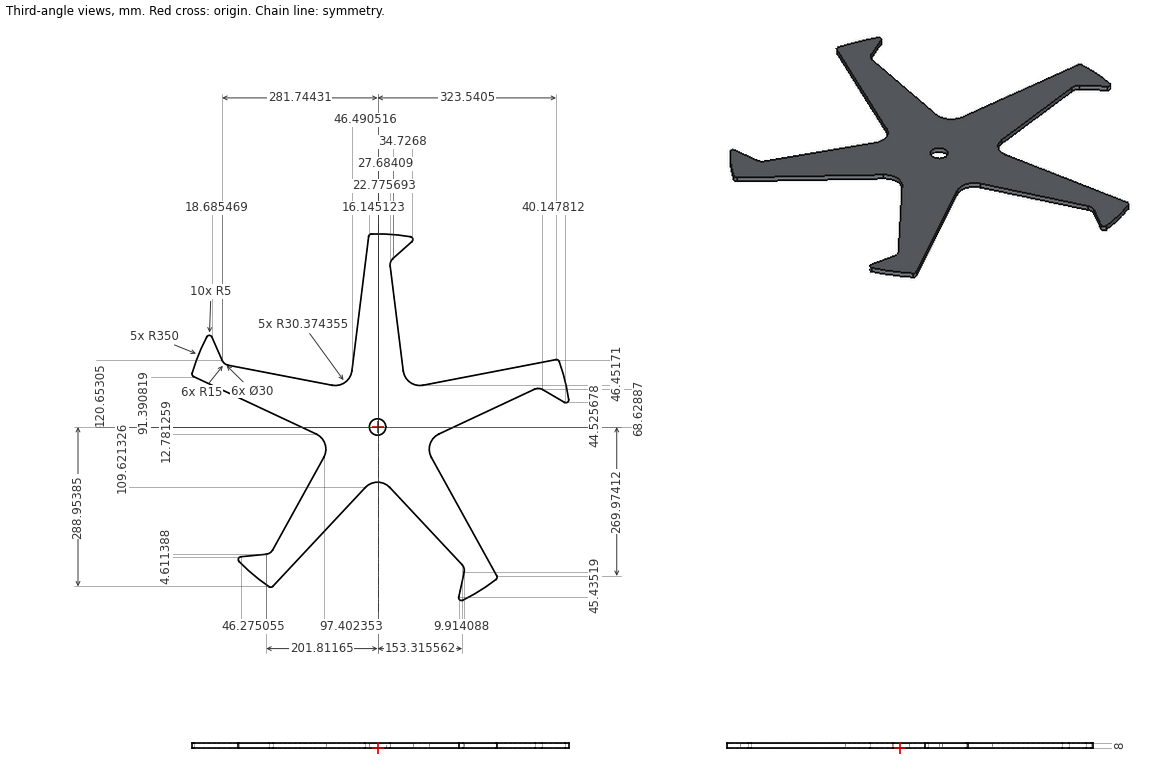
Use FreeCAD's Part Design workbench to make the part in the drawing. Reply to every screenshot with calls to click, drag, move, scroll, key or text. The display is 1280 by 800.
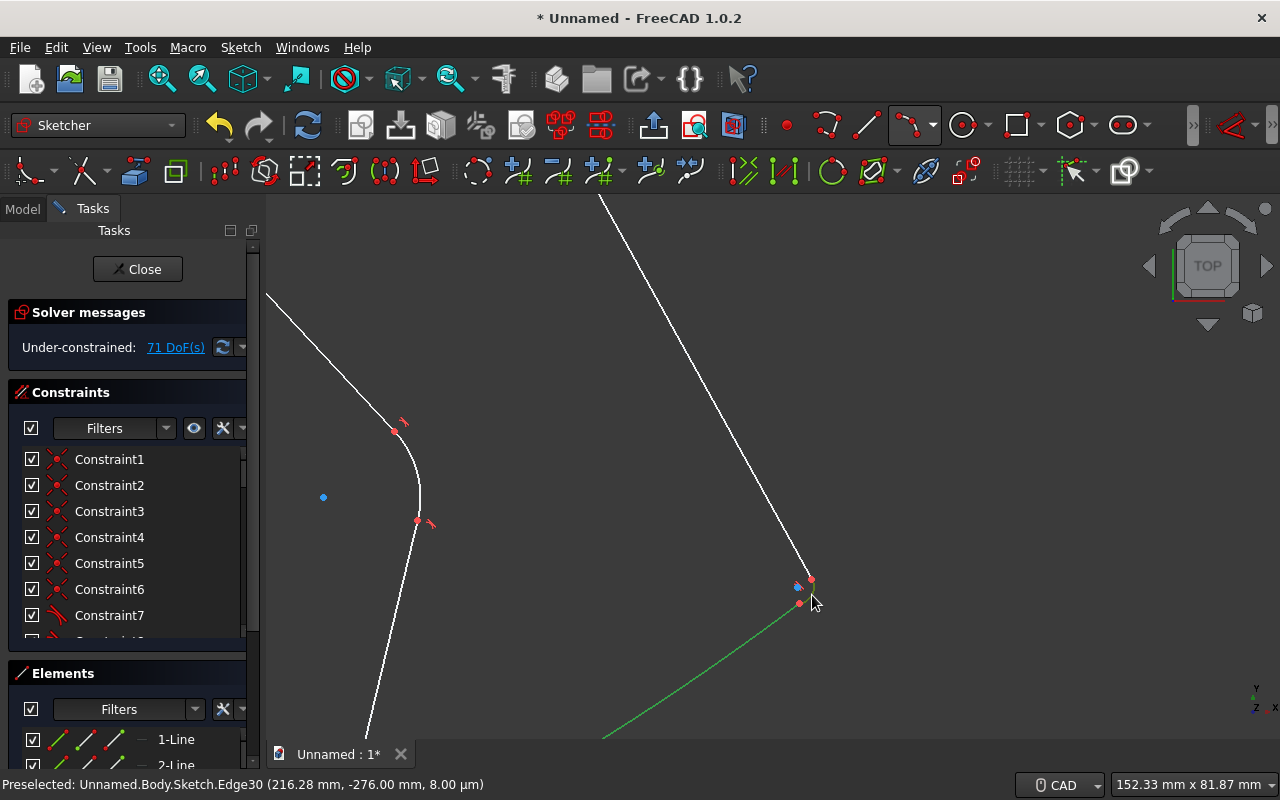
key(t)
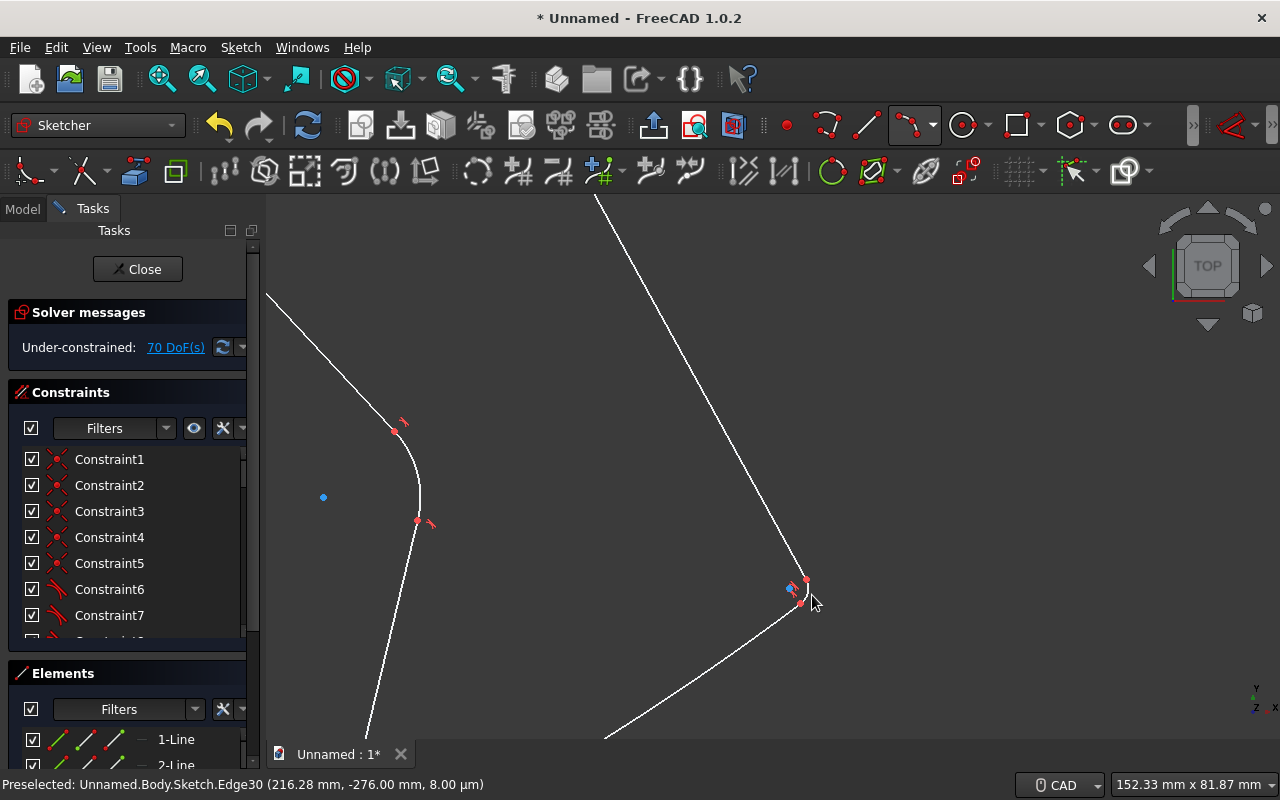
scroll(809, 613, down, 13)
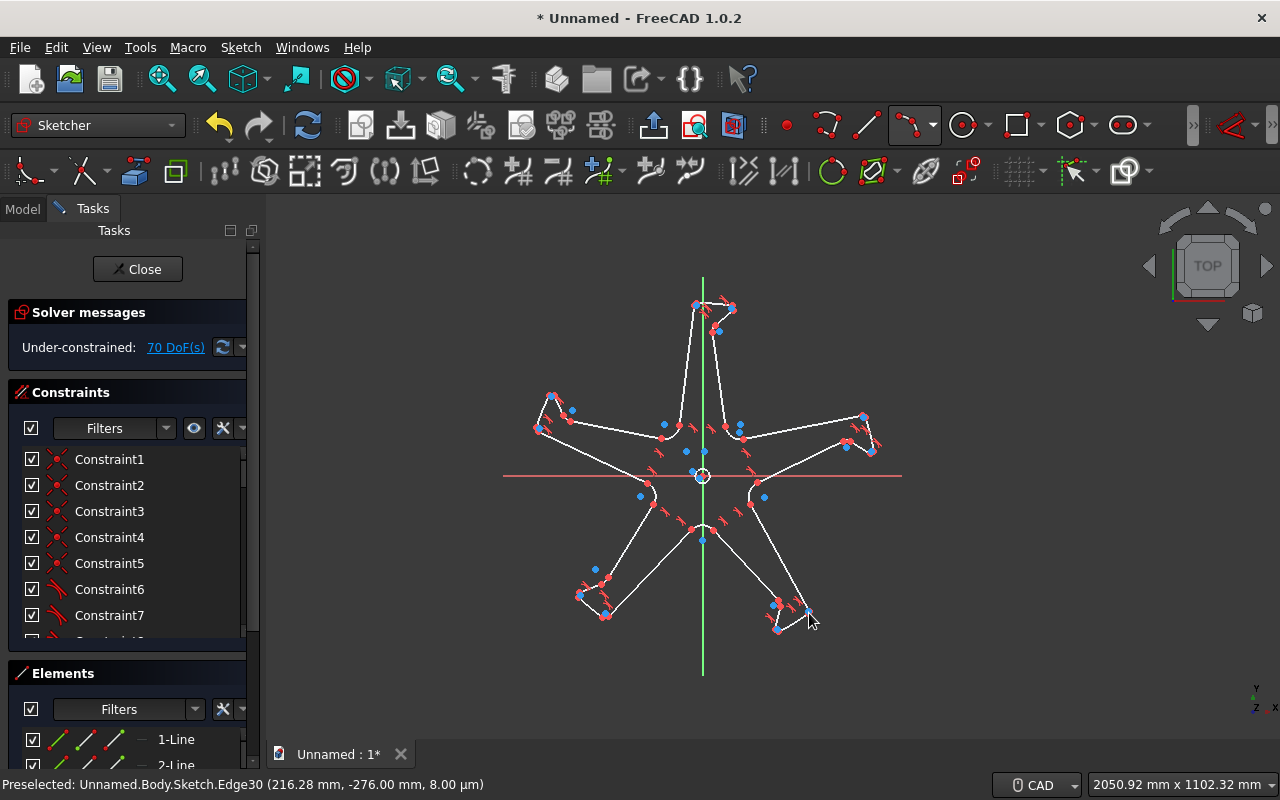
scroll(872, 454, up, 12)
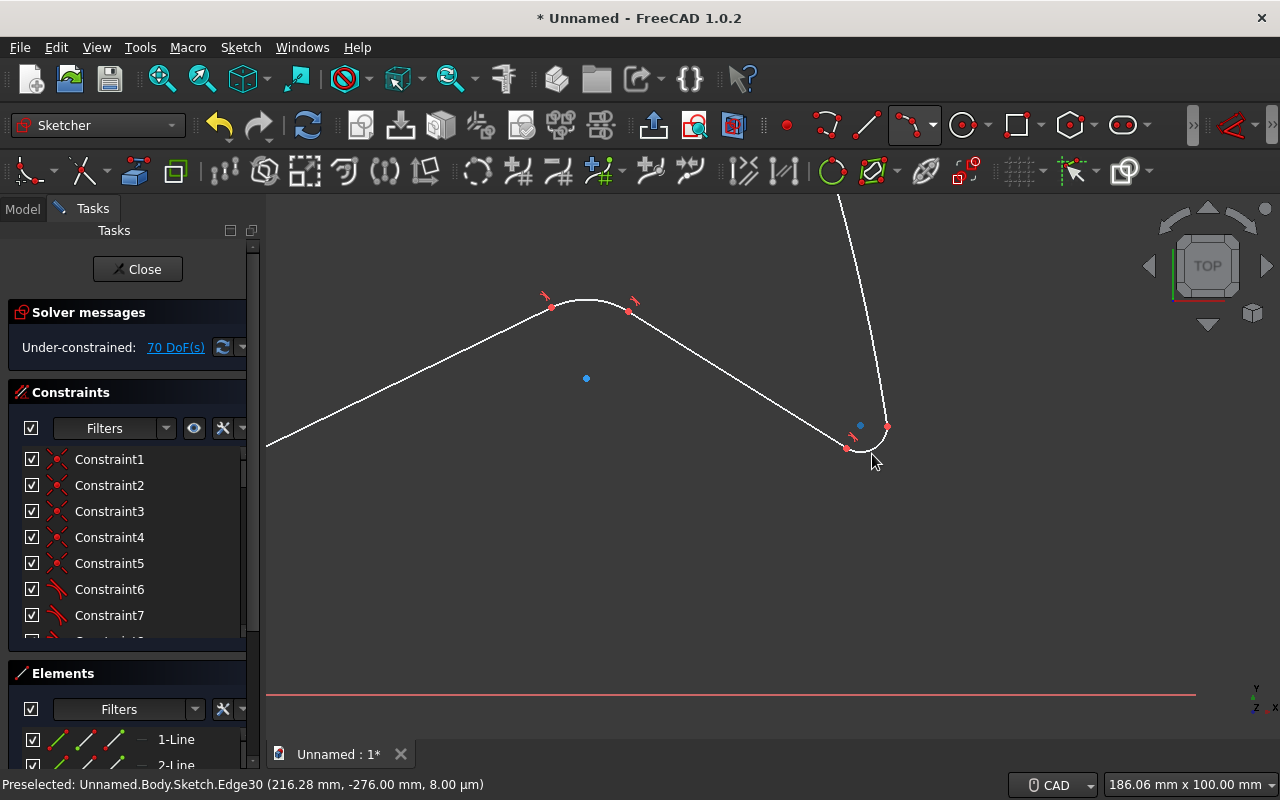
click(863, 452)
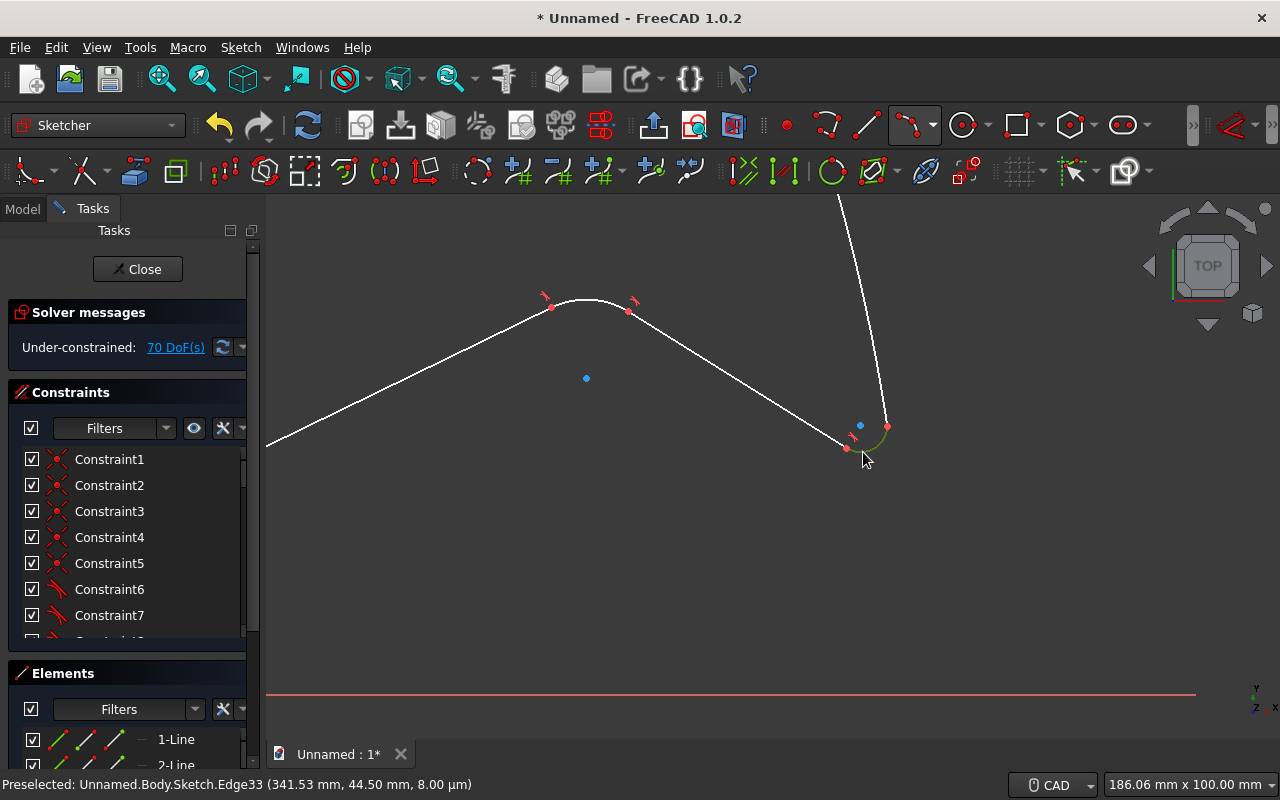
scroll(872, 453, down, 12)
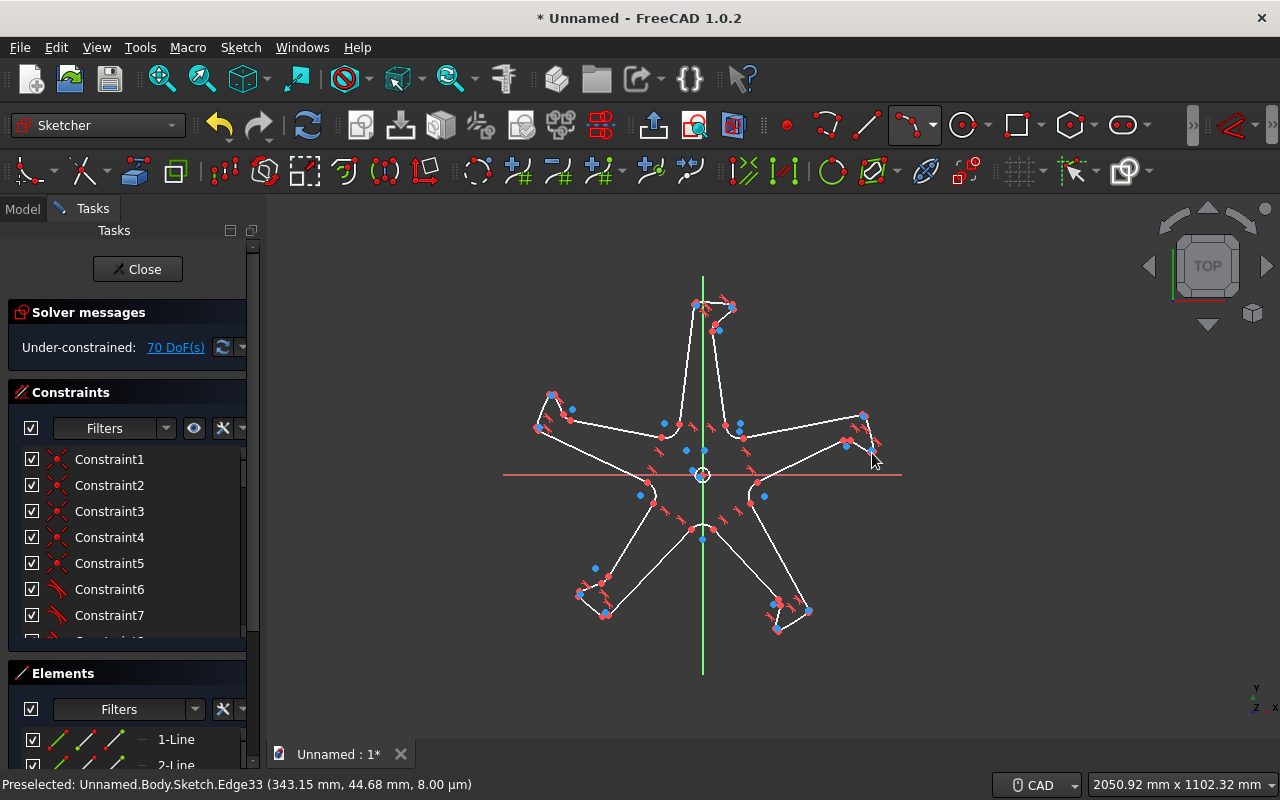
scroll(872, 441, up, 2)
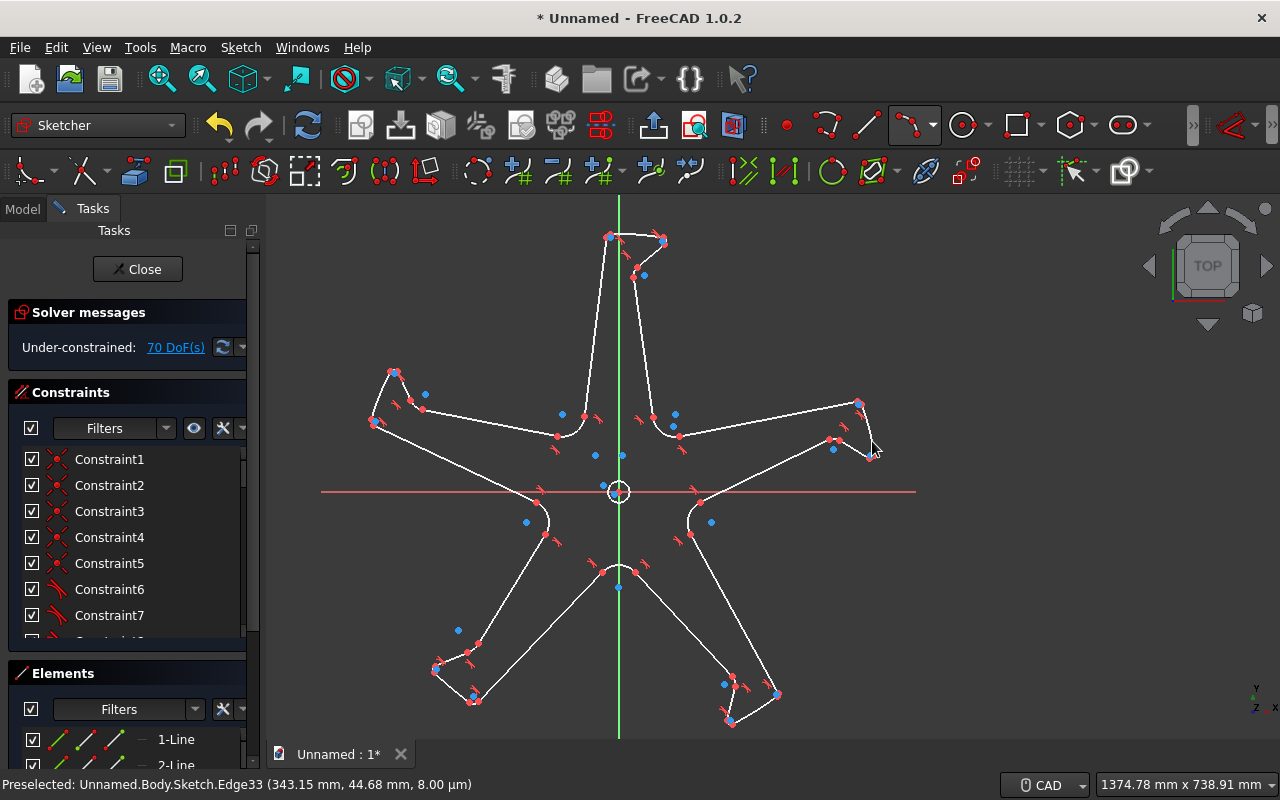
click(872, 440)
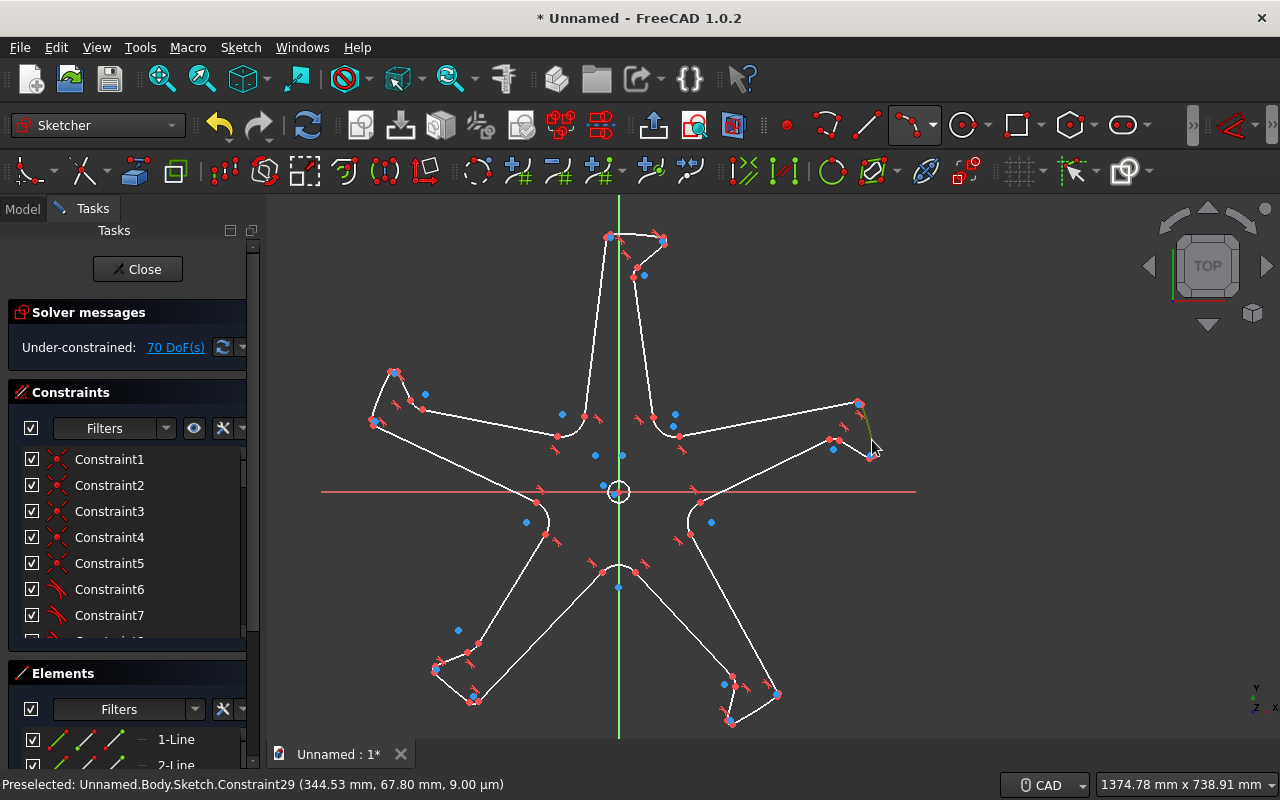
key(t)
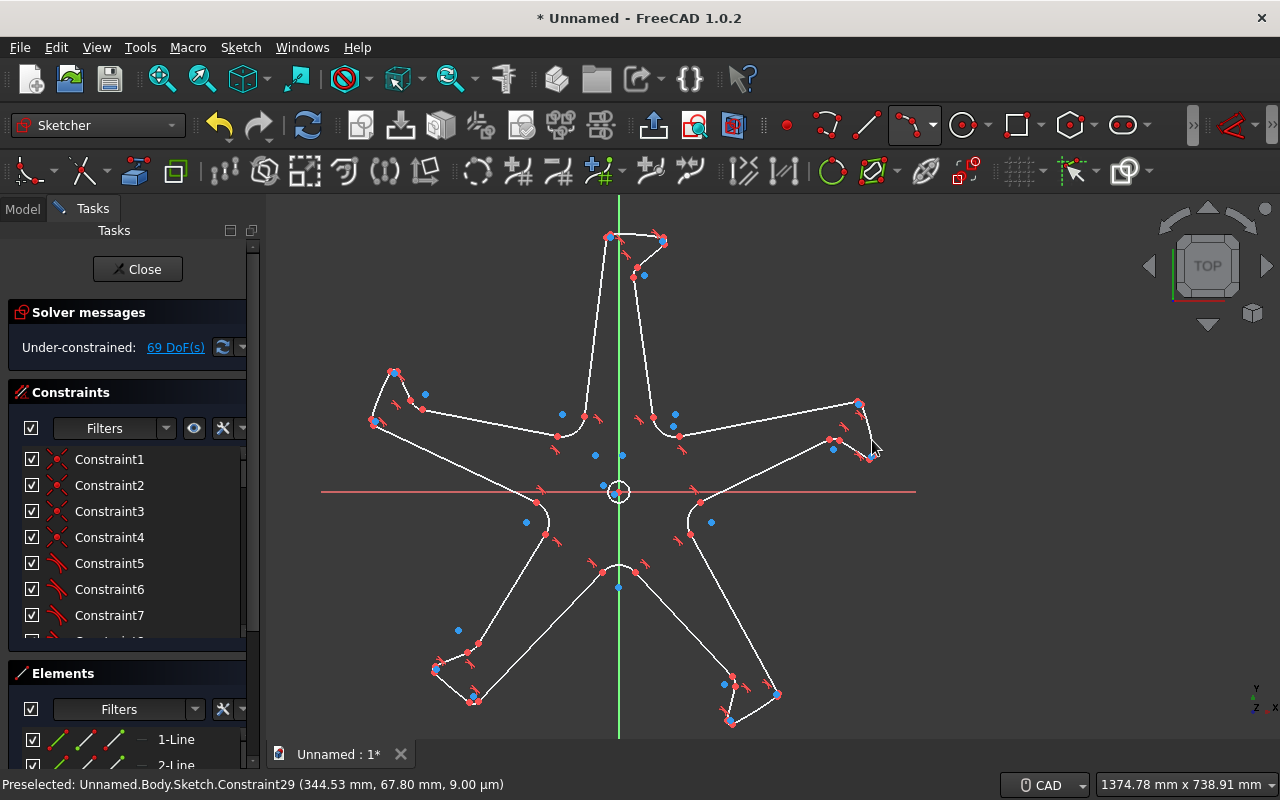
click(872, 440)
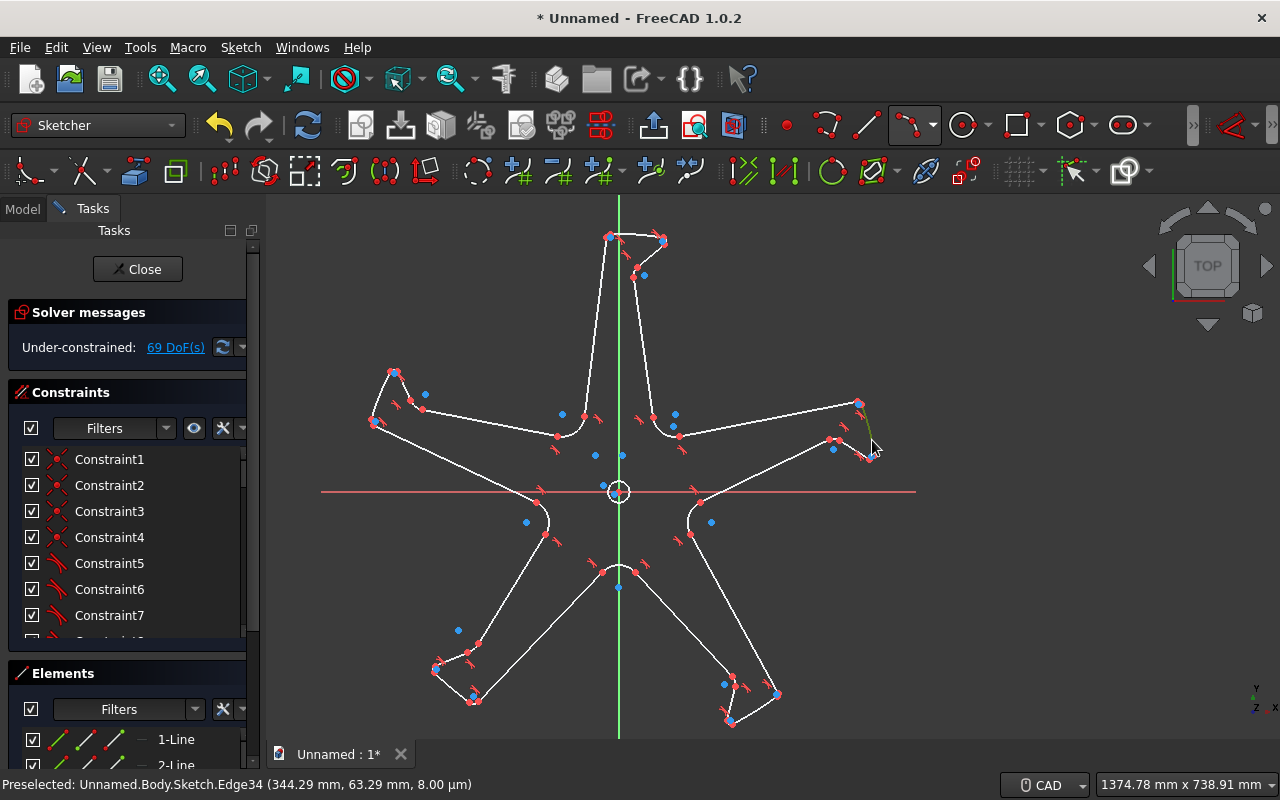
scroll(860, 402, up, 8)